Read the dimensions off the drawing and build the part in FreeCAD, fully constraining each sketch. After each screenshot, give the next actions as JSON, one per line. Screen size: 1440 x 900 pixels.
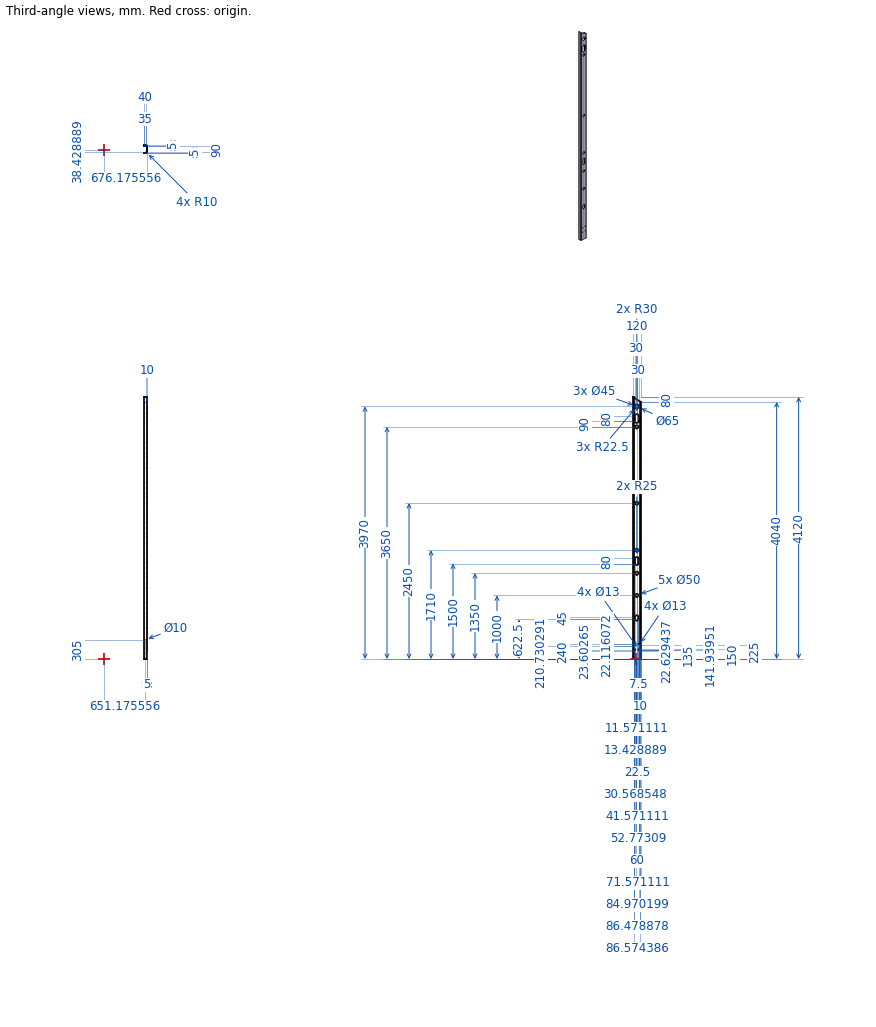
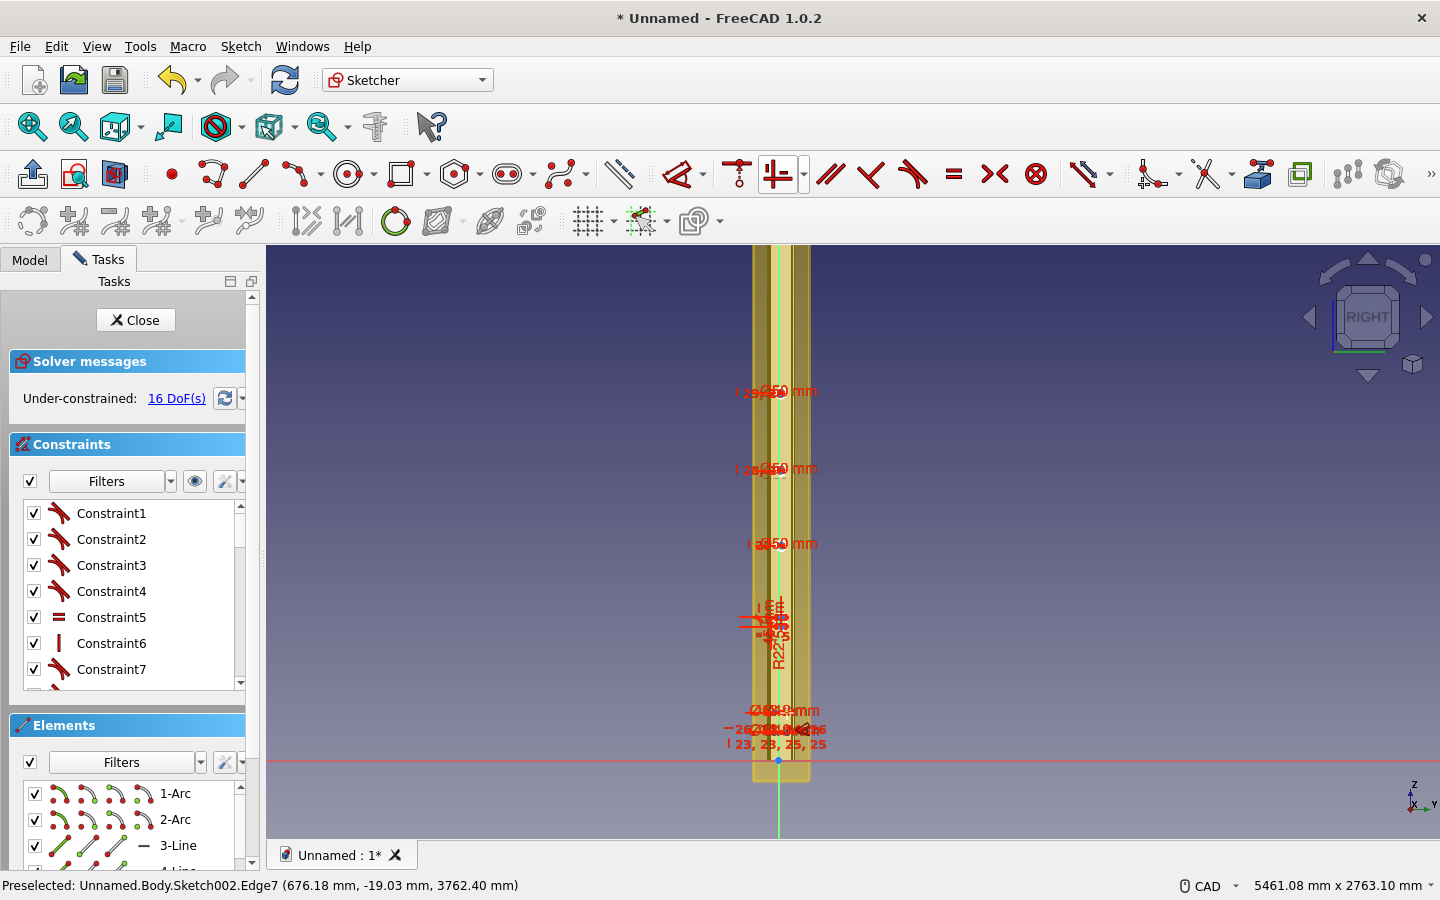
{"action": "left_click", "coordinate": [787, 713]}
{"action": "left_click", "coordinate": [821, 737]}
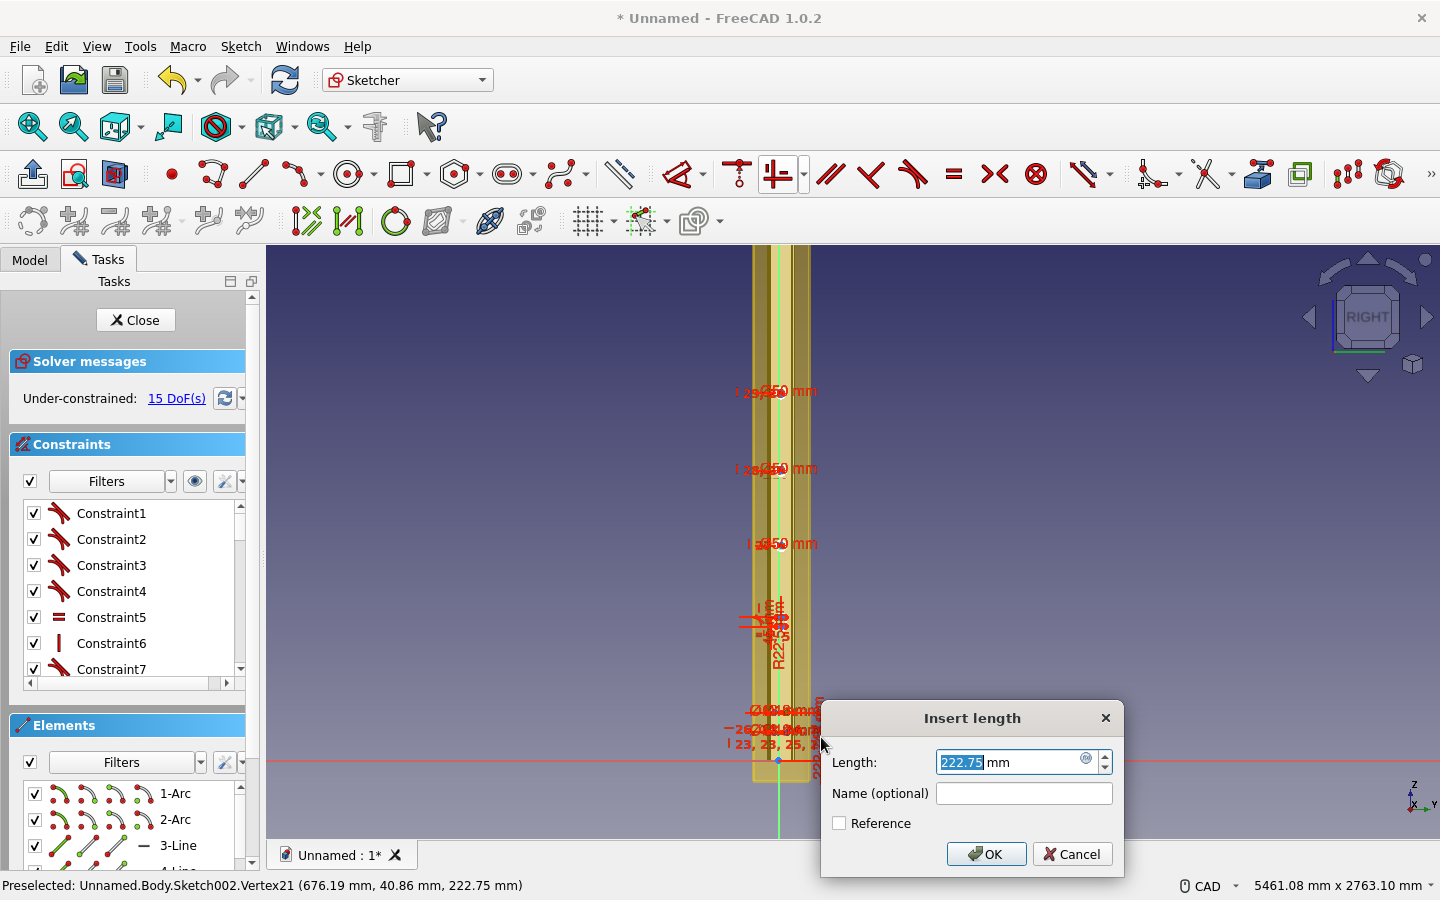
{"action": "type", "text": "225"}
{"action": "key", "text": "Return"}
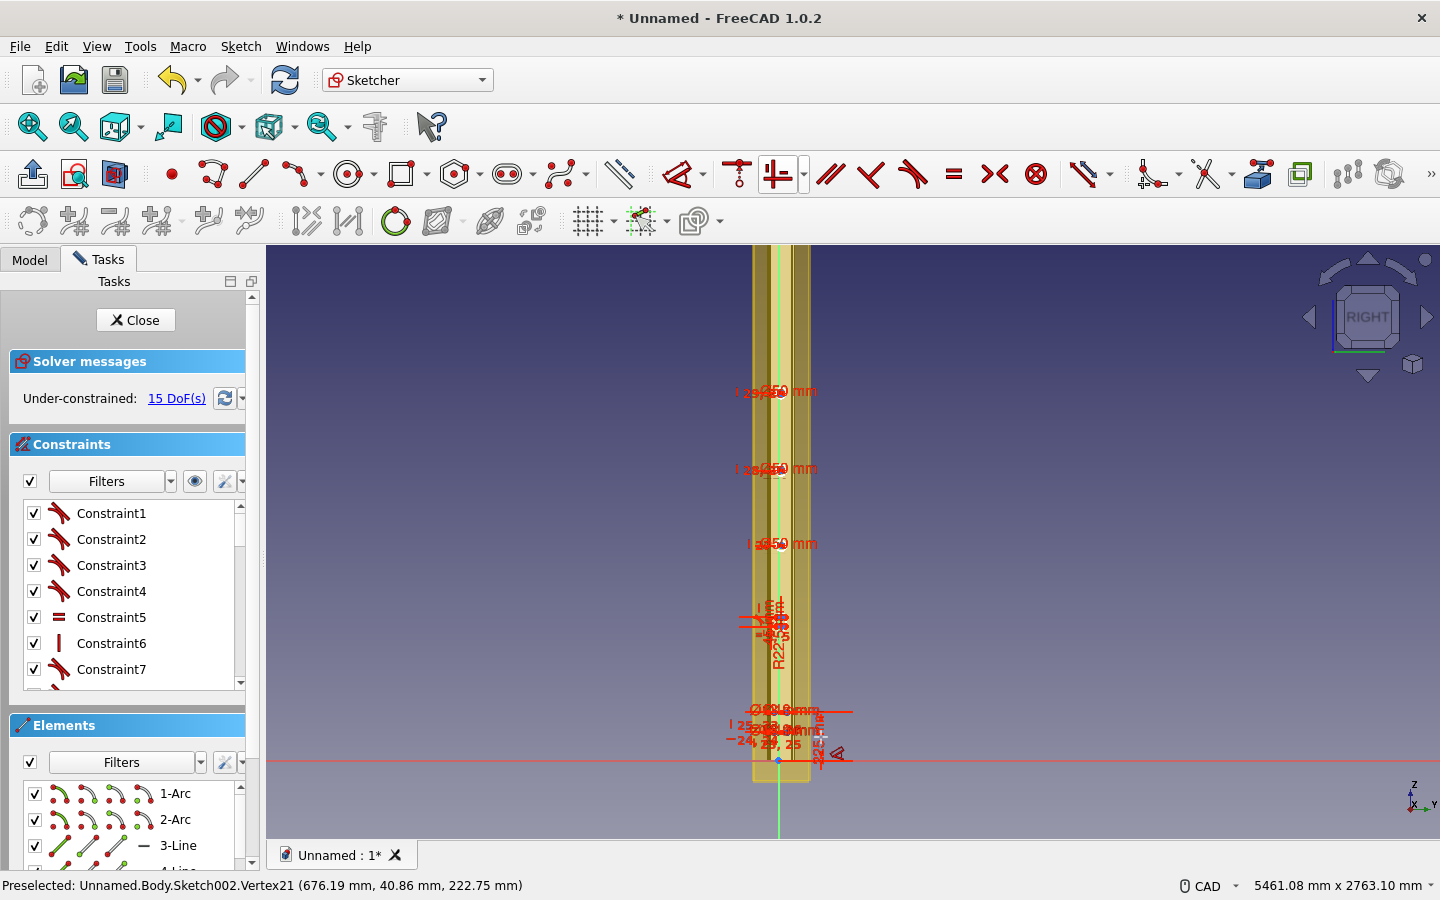
{"action": "scroll", "coordinate": [787, 732], "scroll_direction": "up", "scroll_amount": 2}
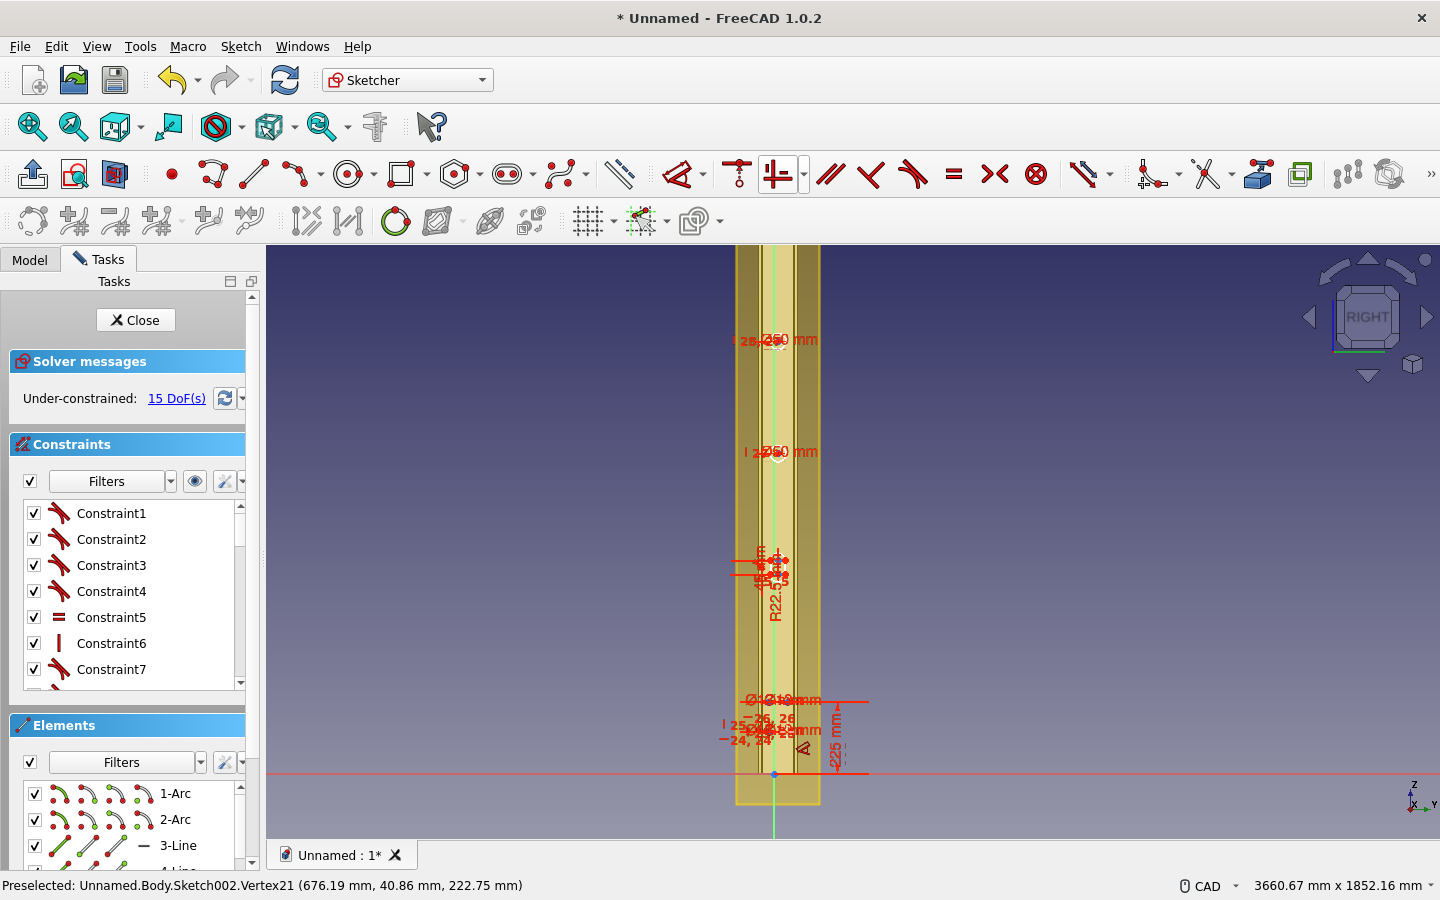
{"action": "left_click", "coordinate": [787, 732]}
{"action": "left_click", "coordinate": [740, 753]}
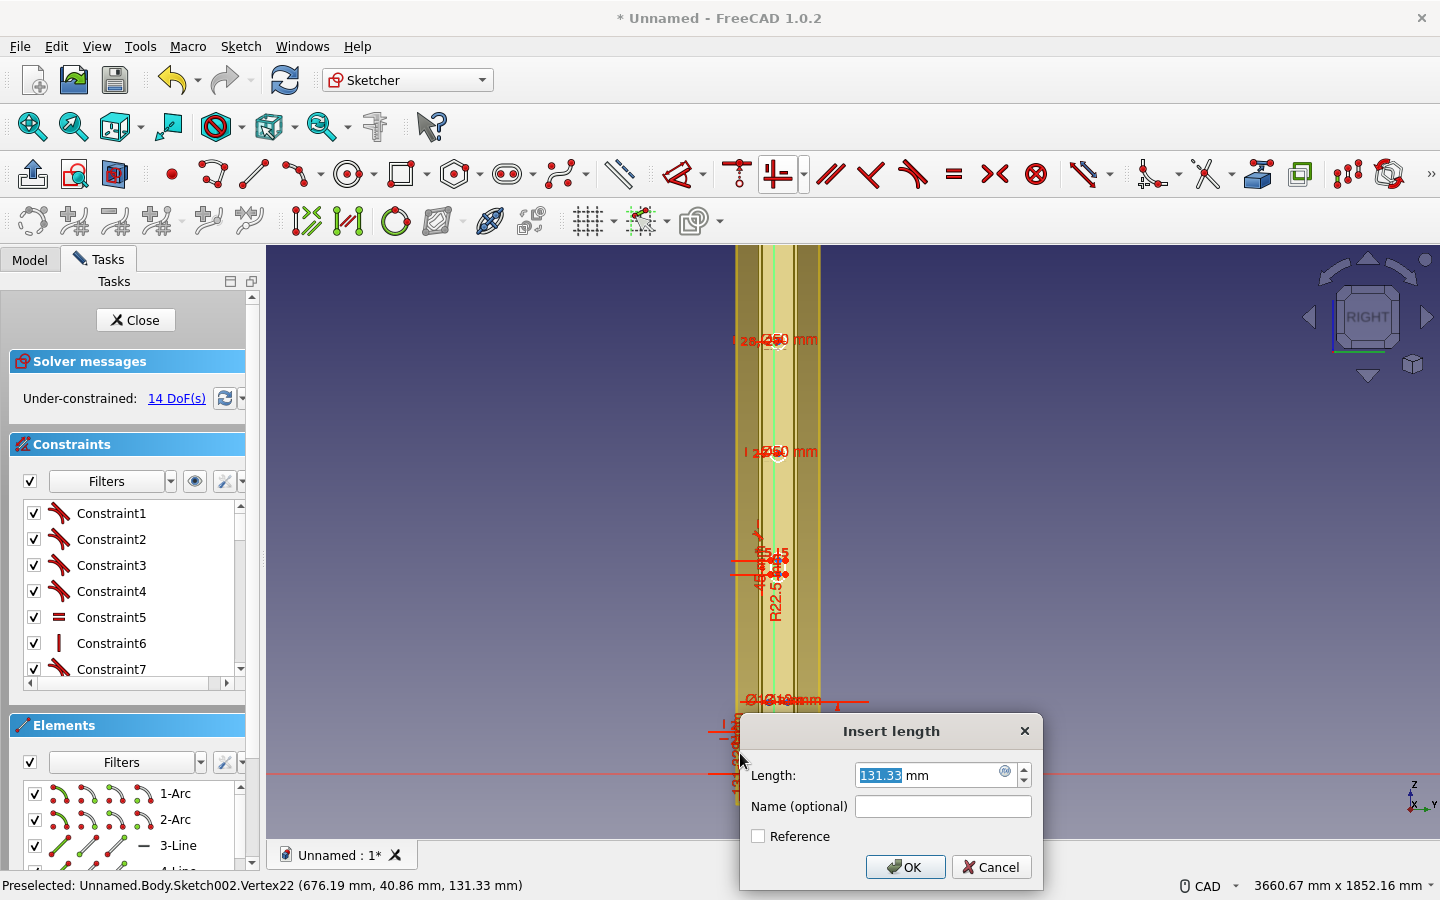
{"action": "type", "text": "135"}
{"action": "key", "text": "Return"}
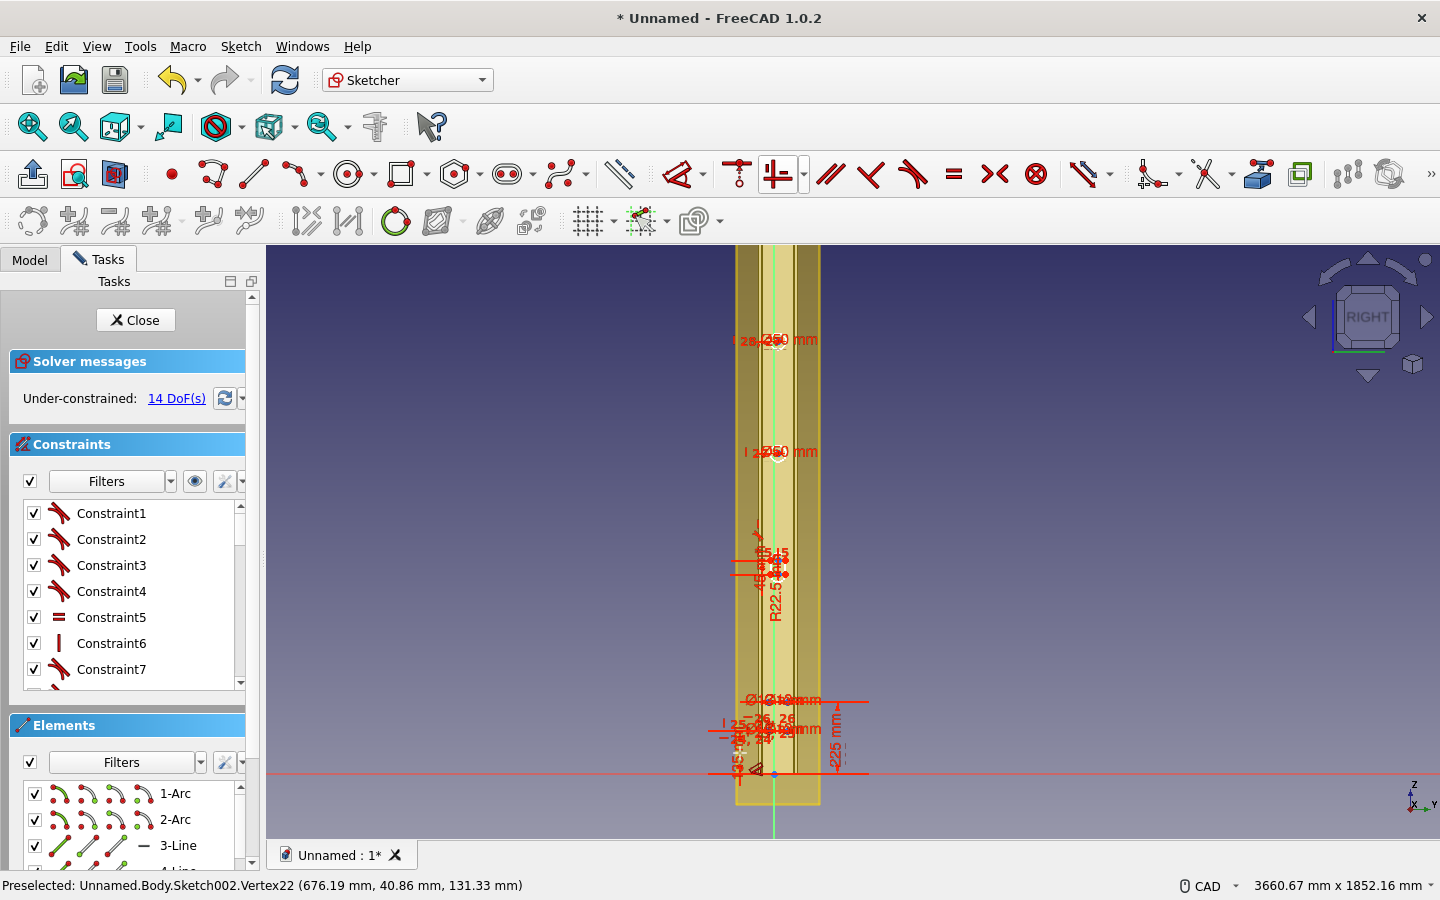
{"action": "scroll", "coordinate": [787, 731], "scroll_direction": "up", "scroll_amount": 4}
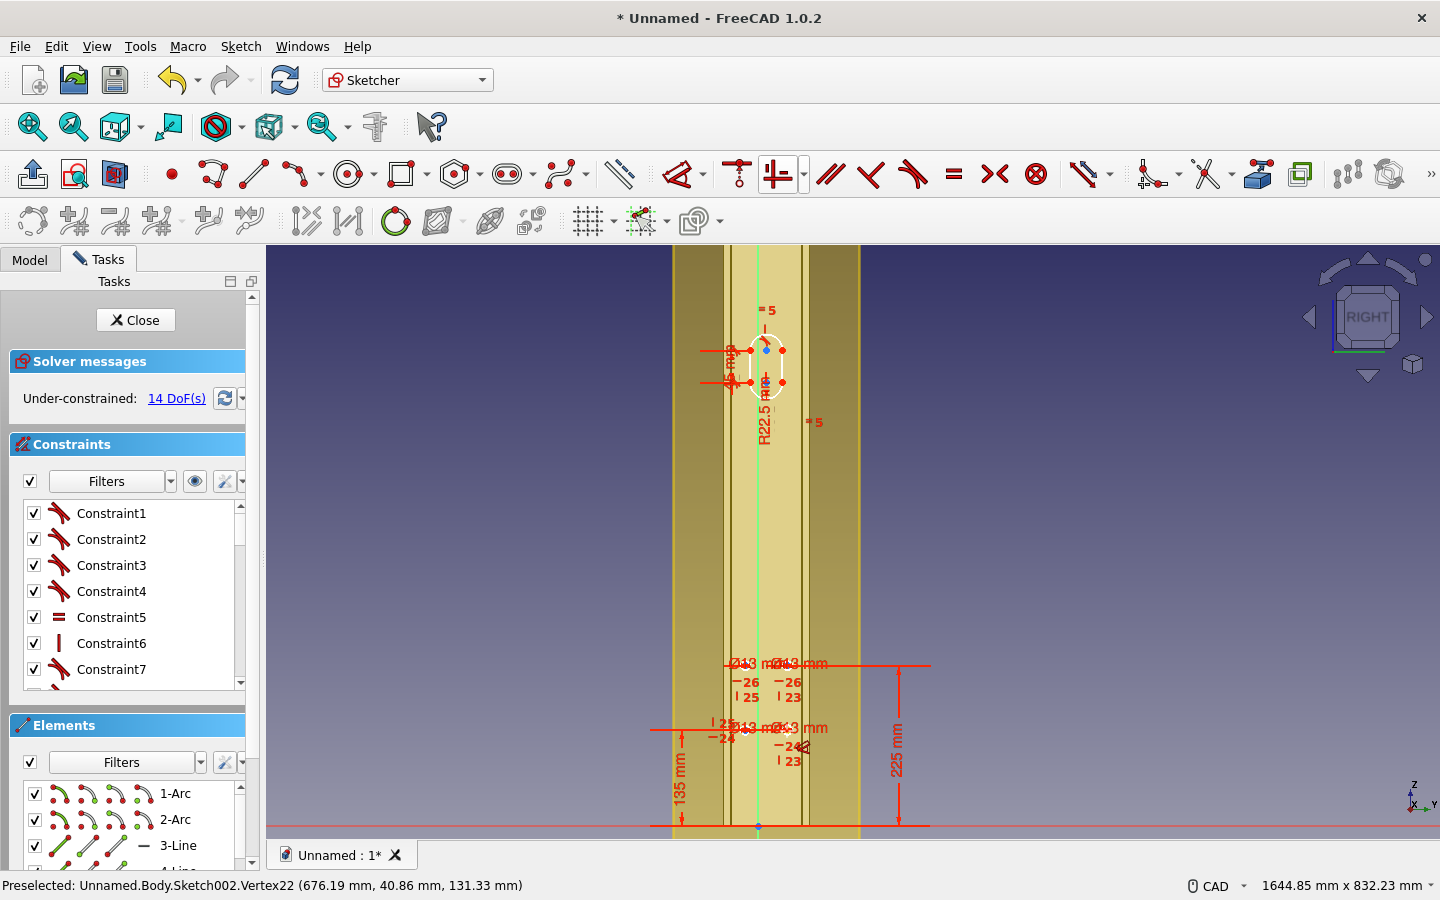
{"action": "left_click", "coordinate": [788, 730]}